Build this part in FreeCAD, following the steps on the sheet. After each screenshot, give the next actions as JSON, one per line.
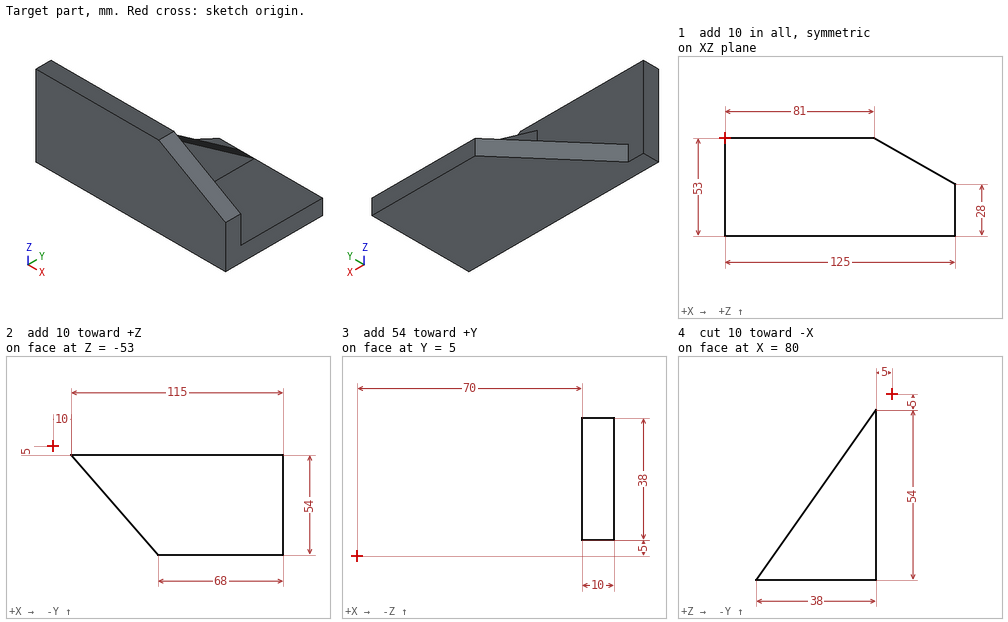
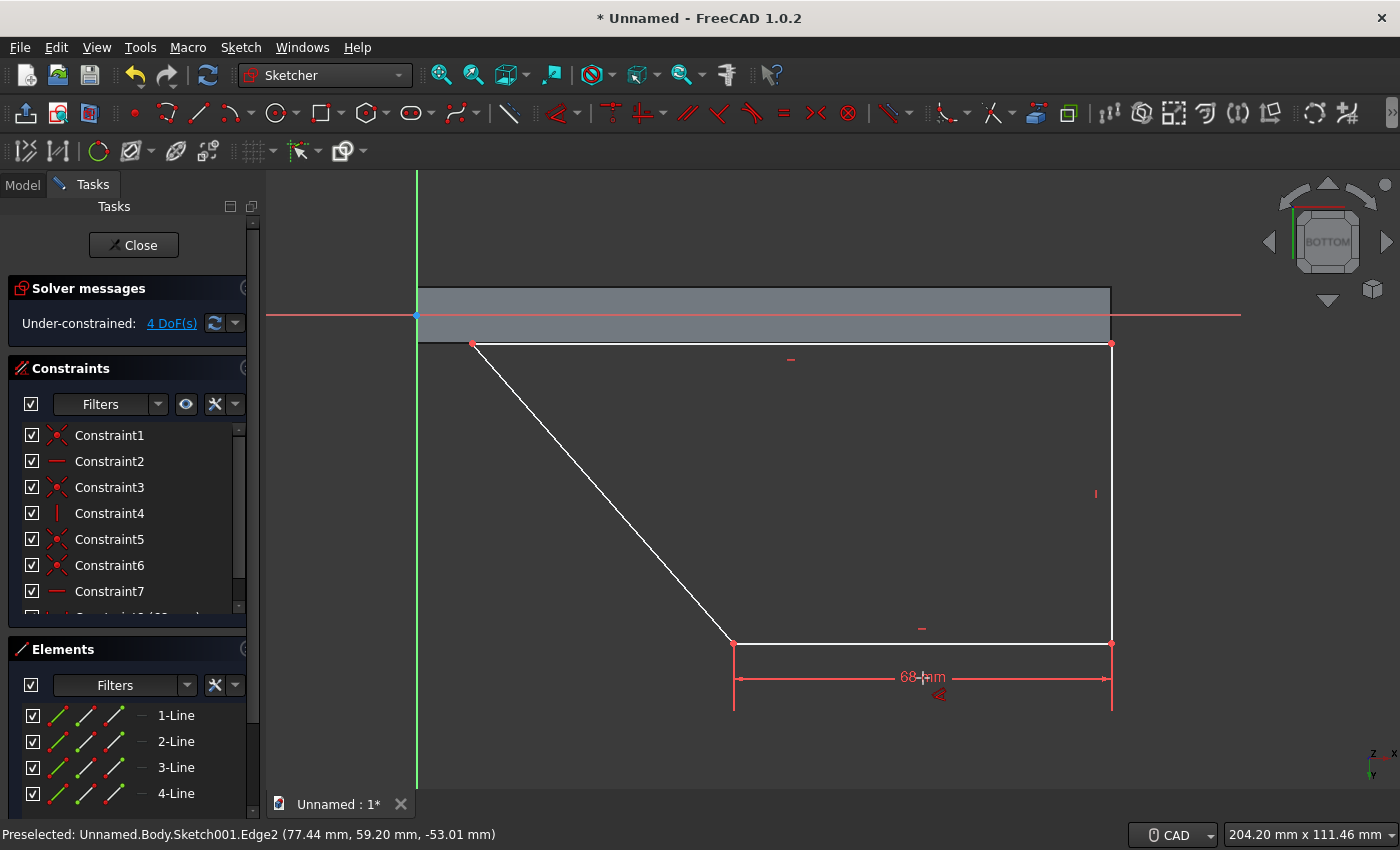
{"action": "left_click", "coordinate": [1112, 554]}
{"action": "left_click", "coordinate": [1146, 494]}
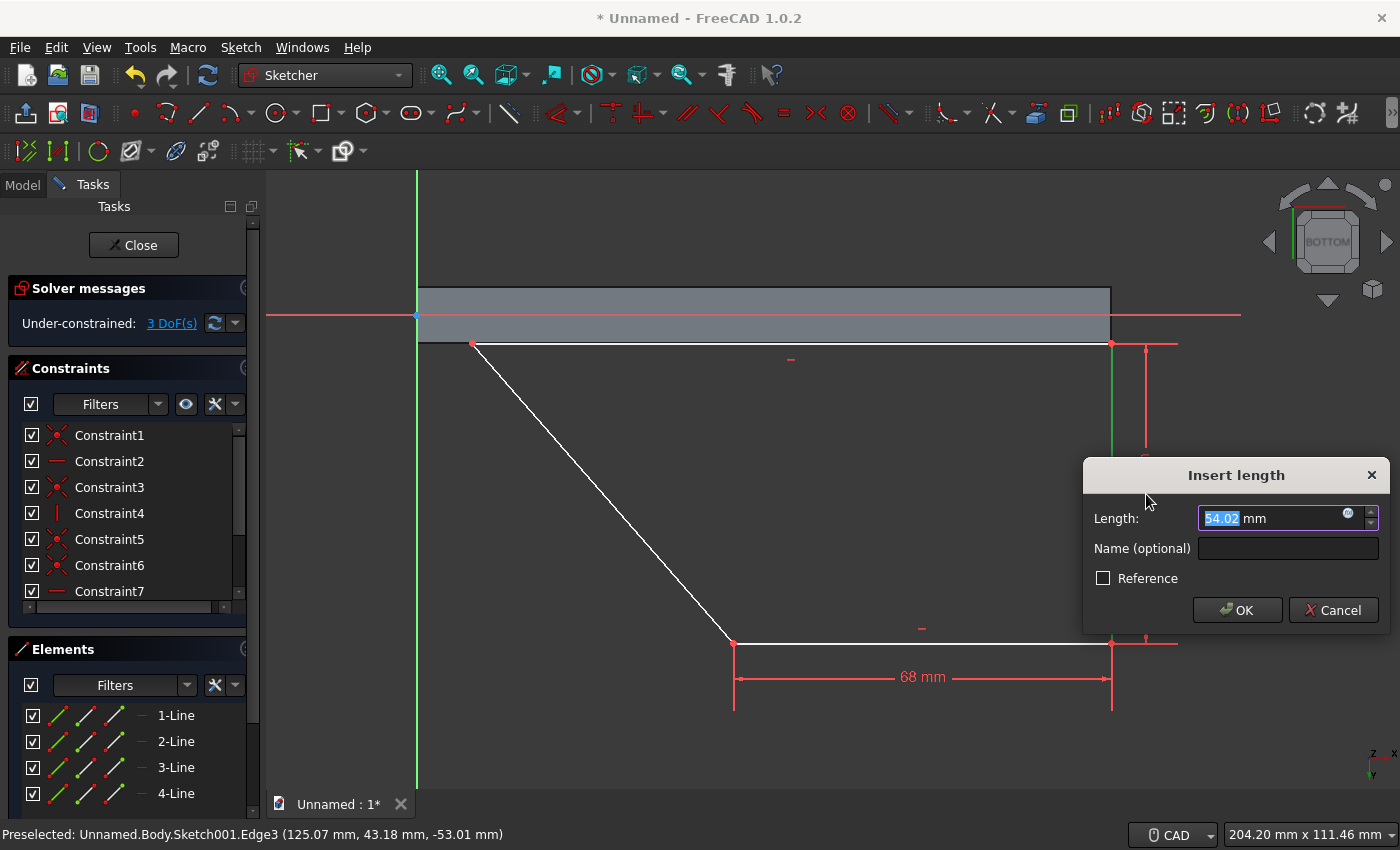
{"action": "type", "text": "54"}
{"action": "key", "text": "Return"}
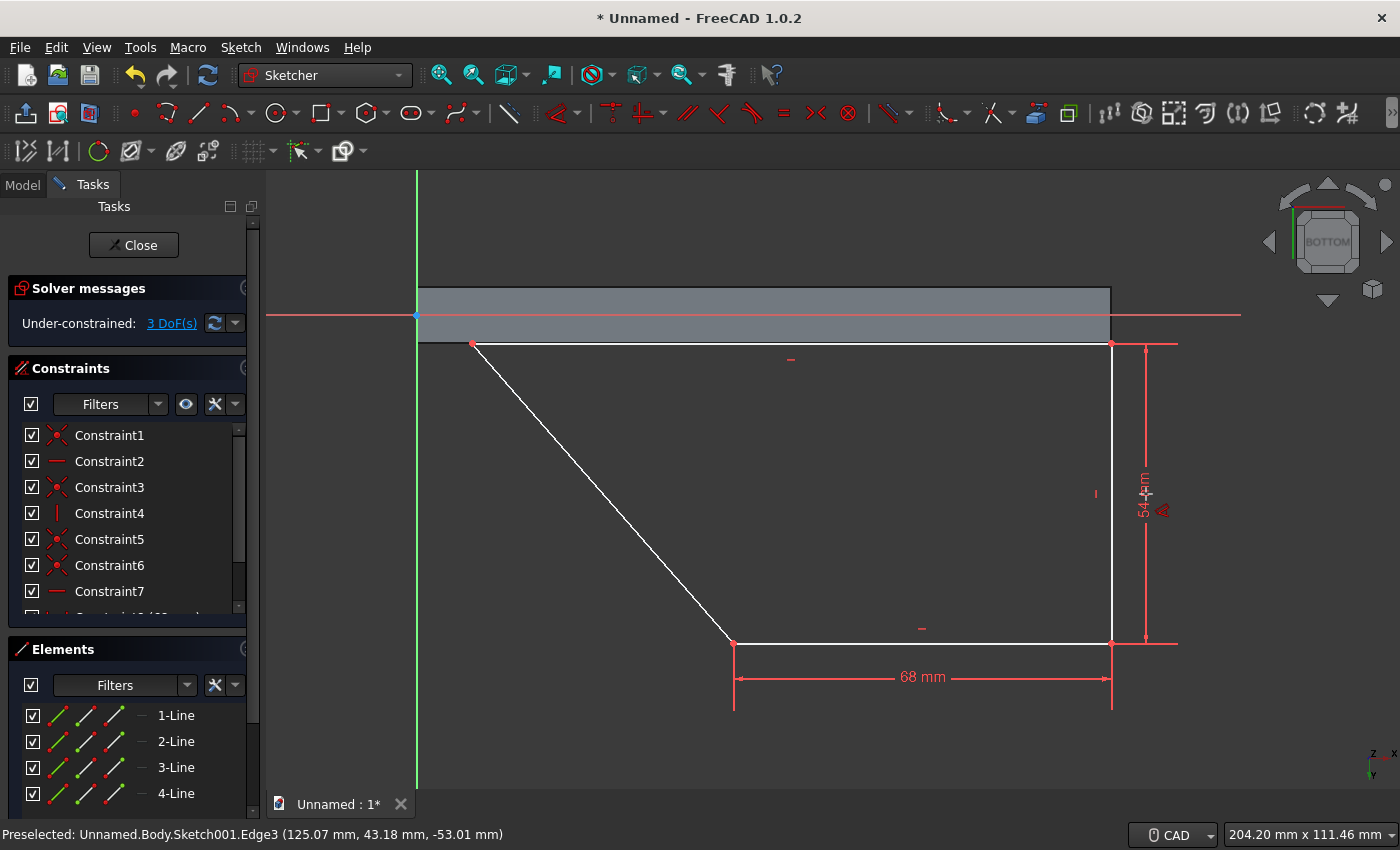
{"action": "scroll", "coordinate": [472, 344], "scroll_direction": "up", "scroll_amount": 2}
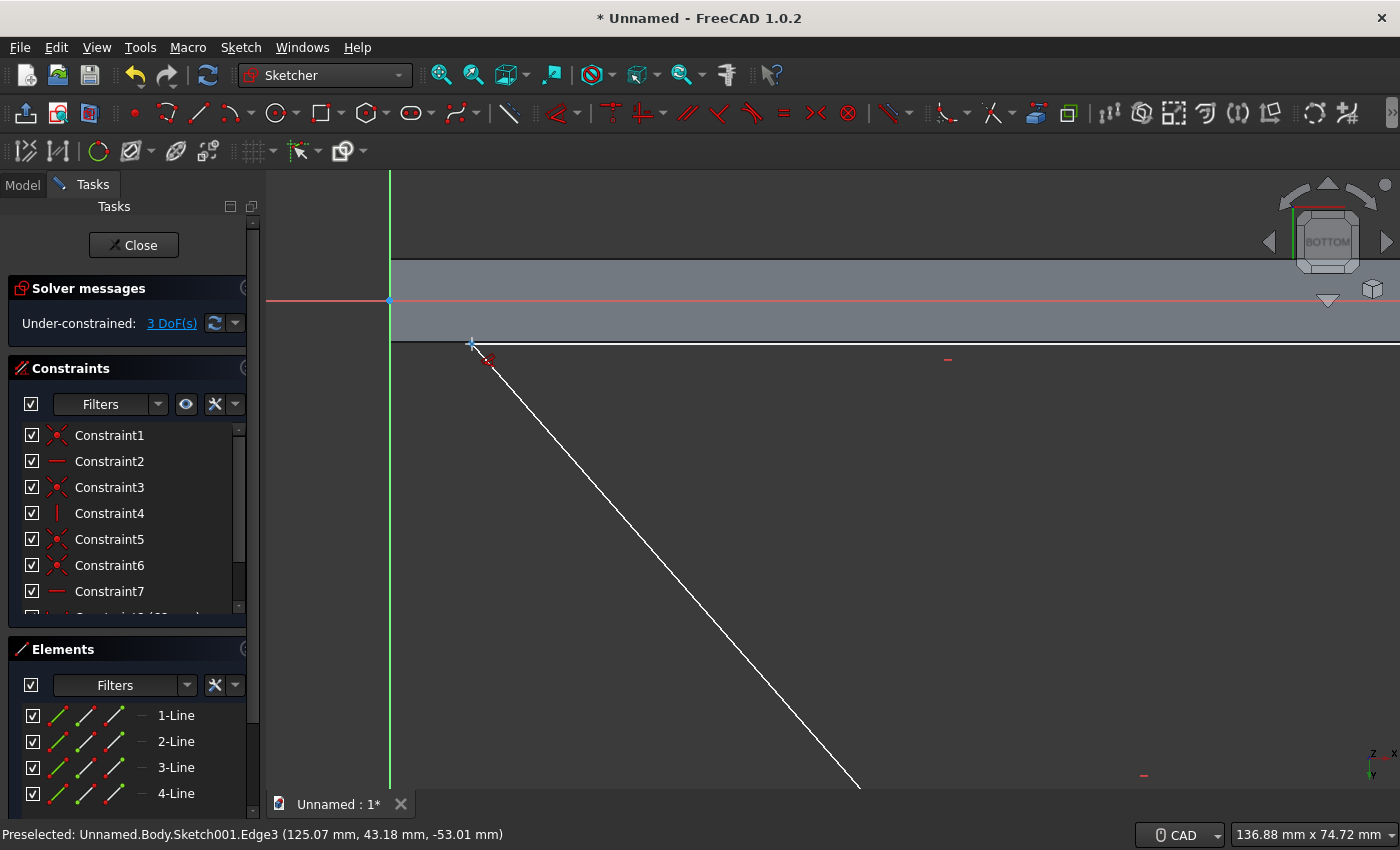
{"action": "left_click", "coordinate": [472, 344]}
{"action": "left_click", "coordinate": [356, 322]}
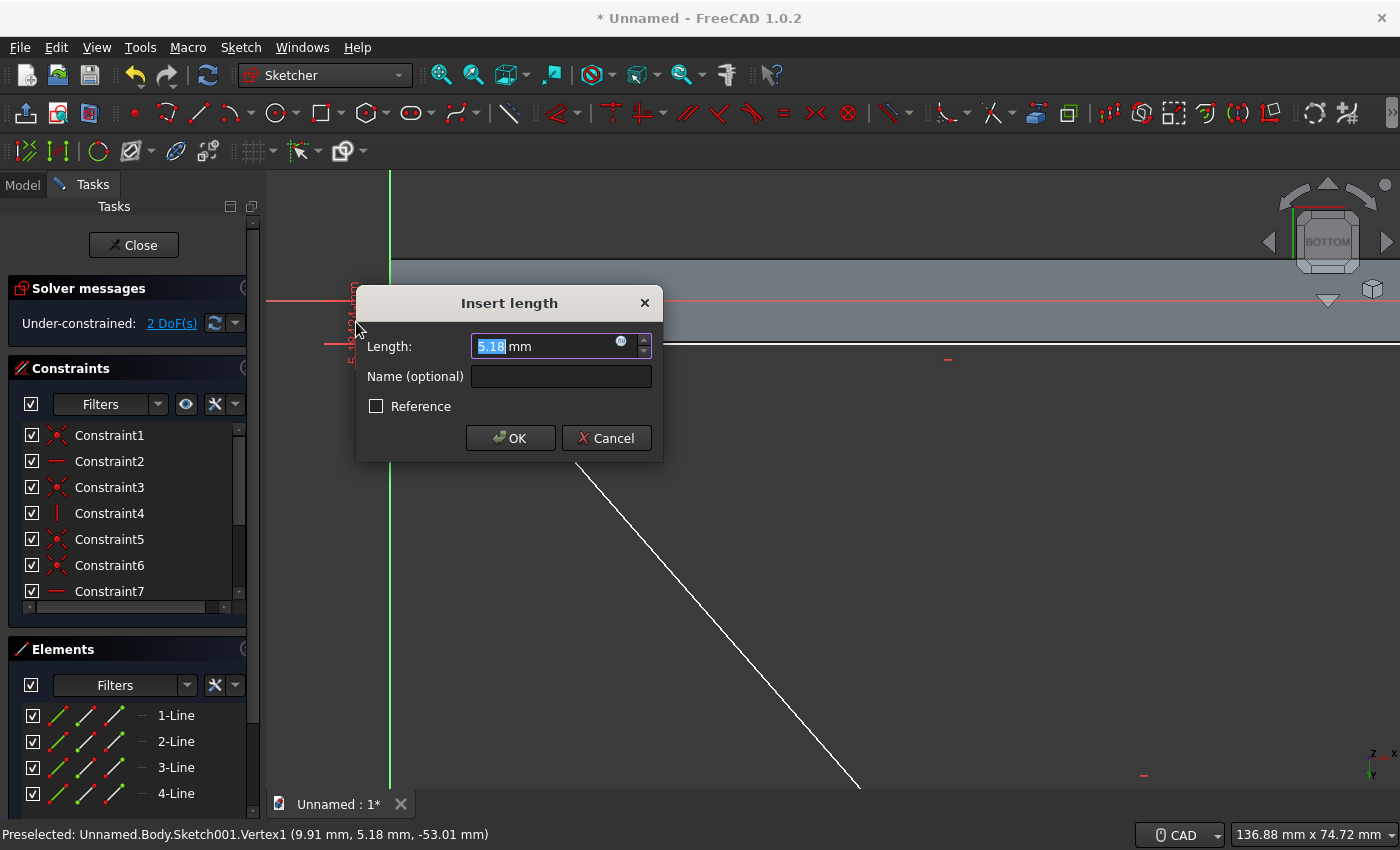
{"action": "type", "text": "5"}
{"action": "key", "text": "Return"}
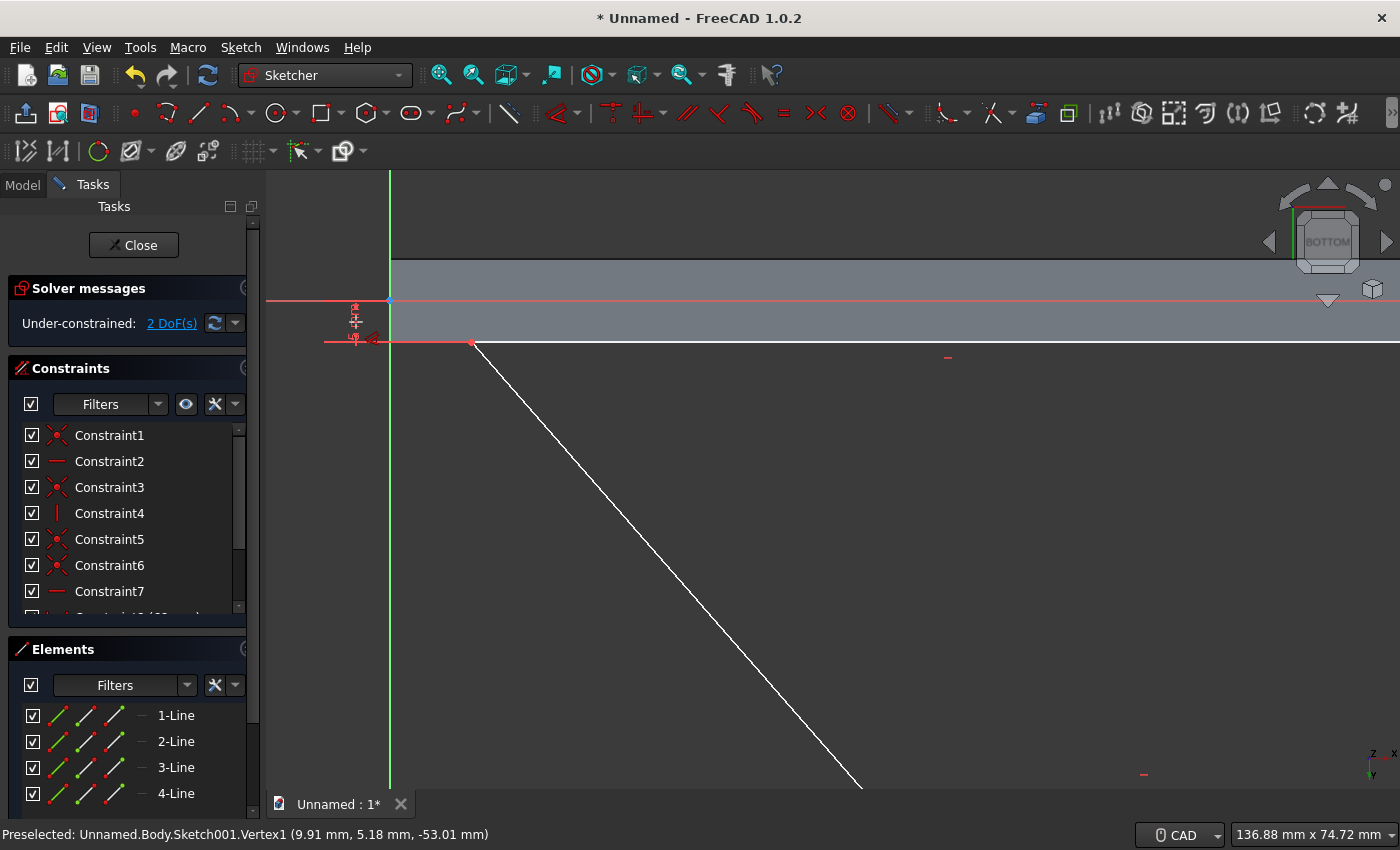
{"action": "left_click", "coordinate": [1140, 342]}
{"action": "left_click", "coordinate": [853, 376]}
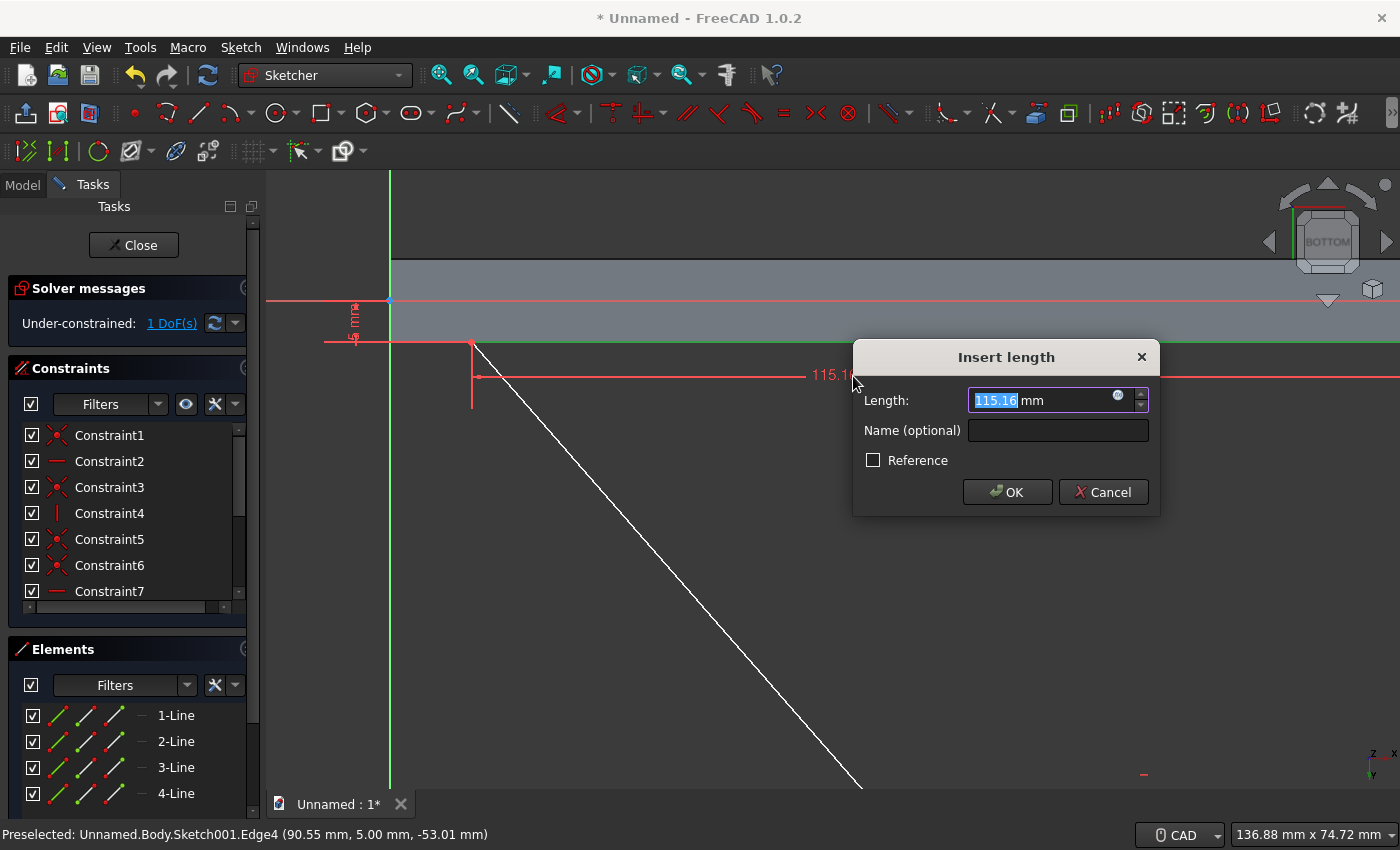
{"action": "type", "text": "115"}
{"action": "key", "text": "Return"}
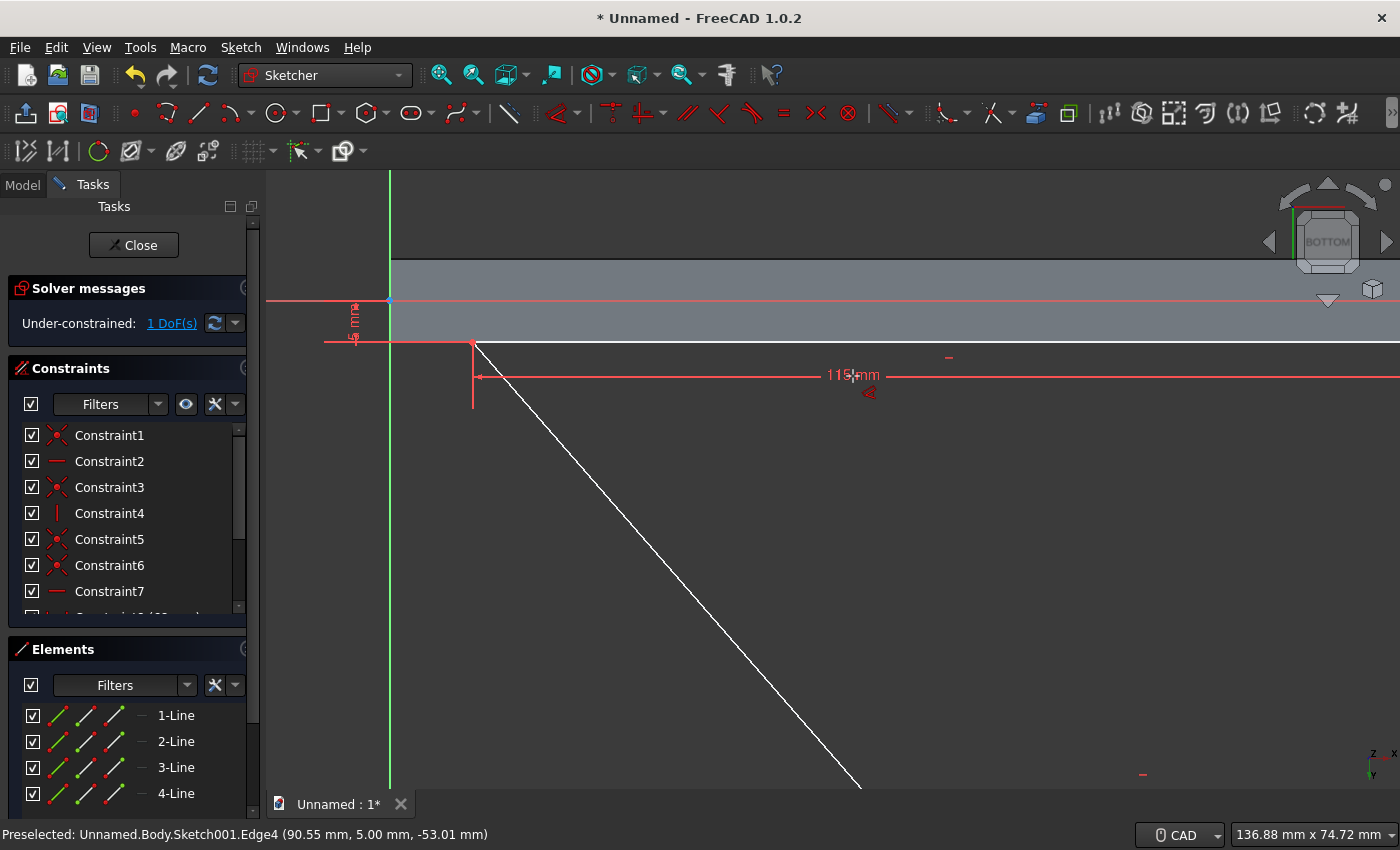
{"action": "left_click", "coordinate": [473, 342]}
{"action": "left_click", "coordinate": [431, 267]}